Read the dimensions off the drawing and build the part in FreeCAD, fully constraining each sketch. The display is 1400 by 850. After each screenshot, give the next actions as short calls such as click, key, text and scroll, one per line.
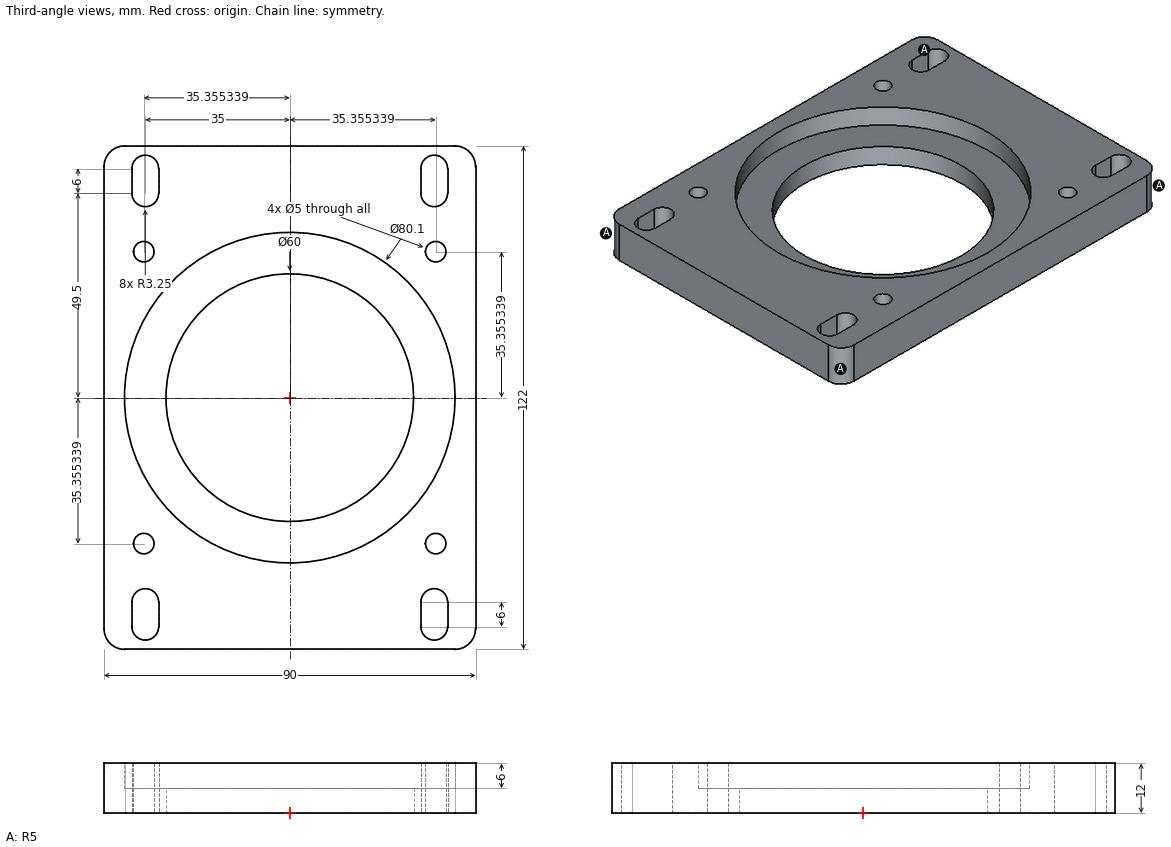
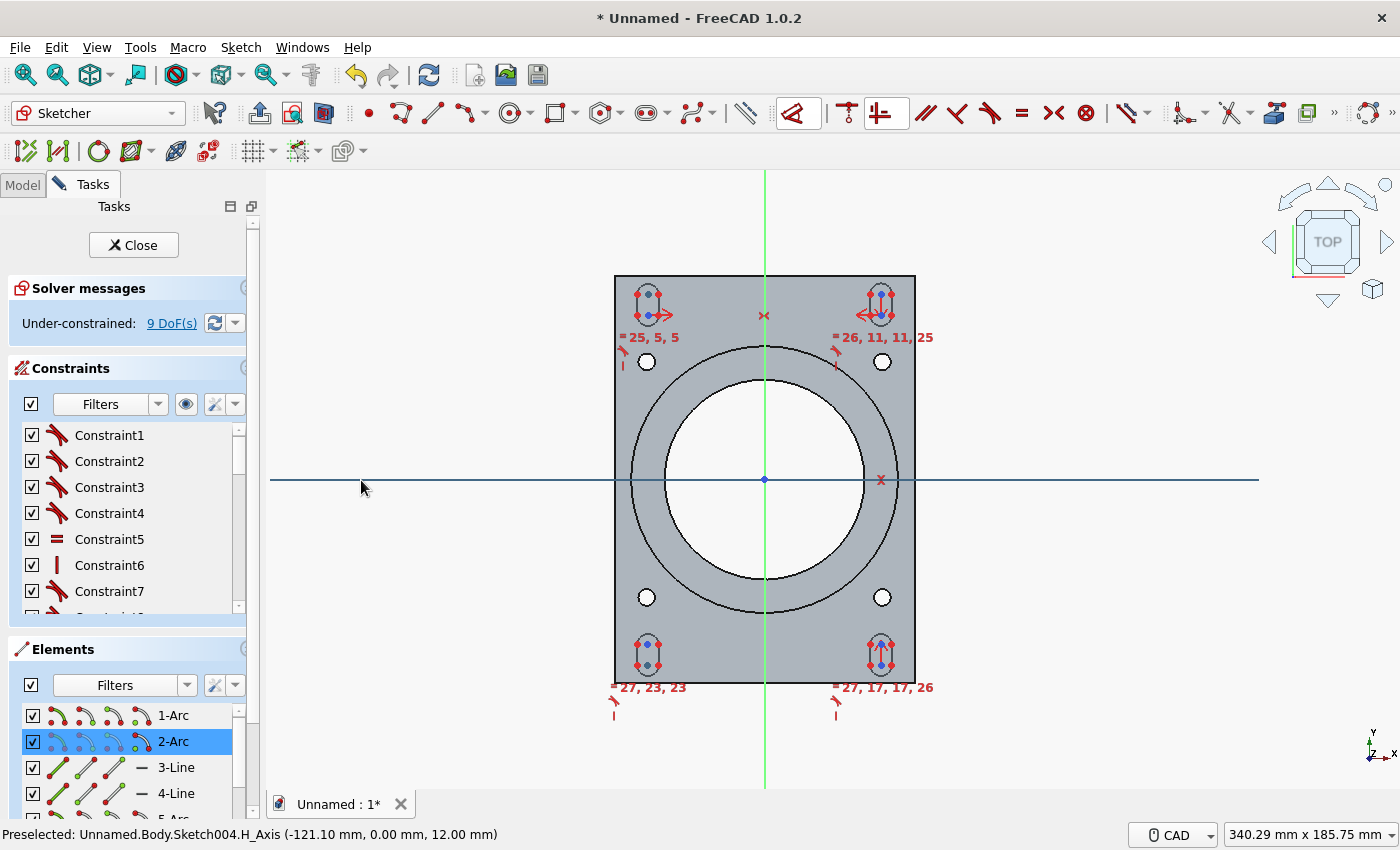
click(1054, 114)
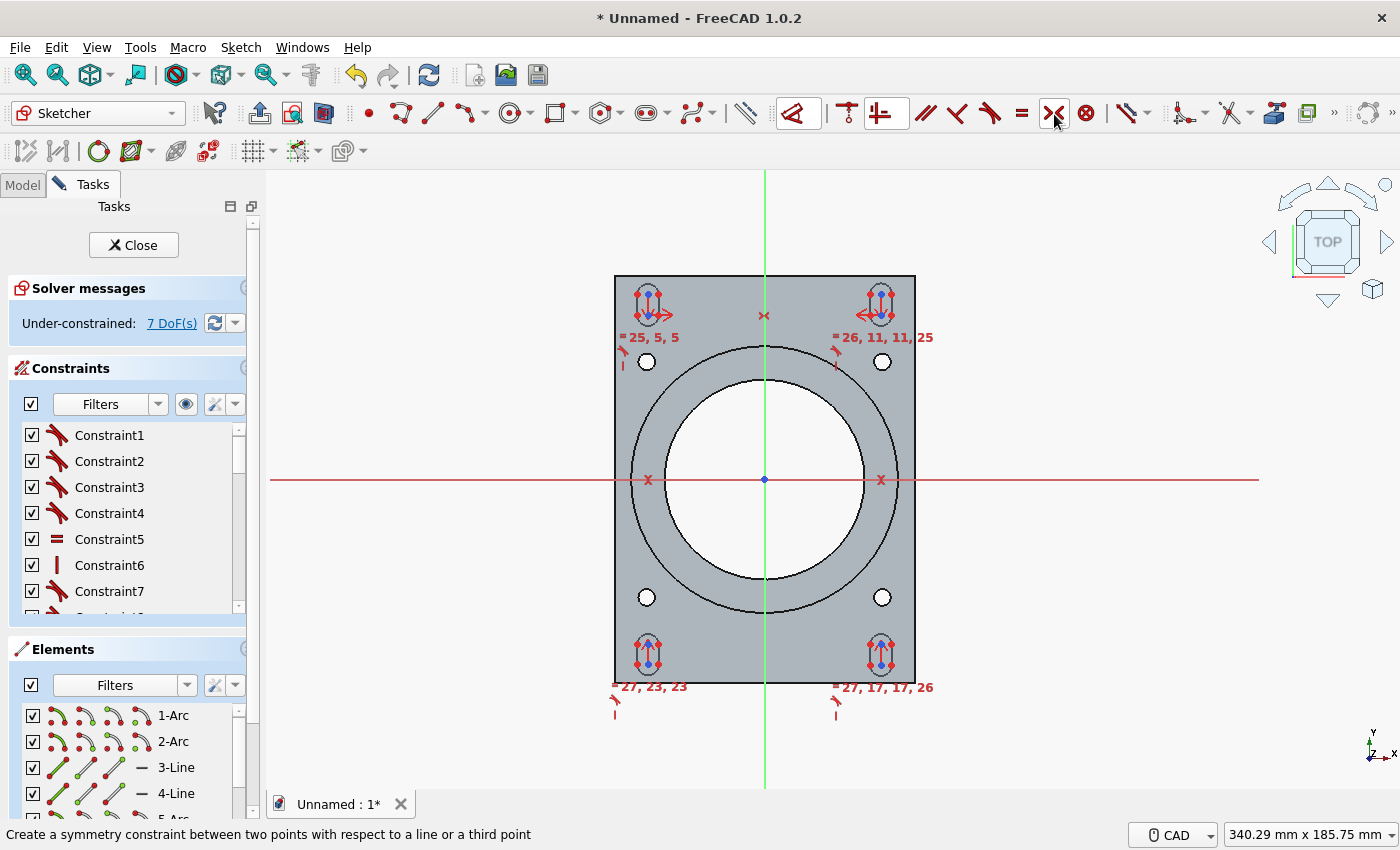
scroll(642, 324, up, 7)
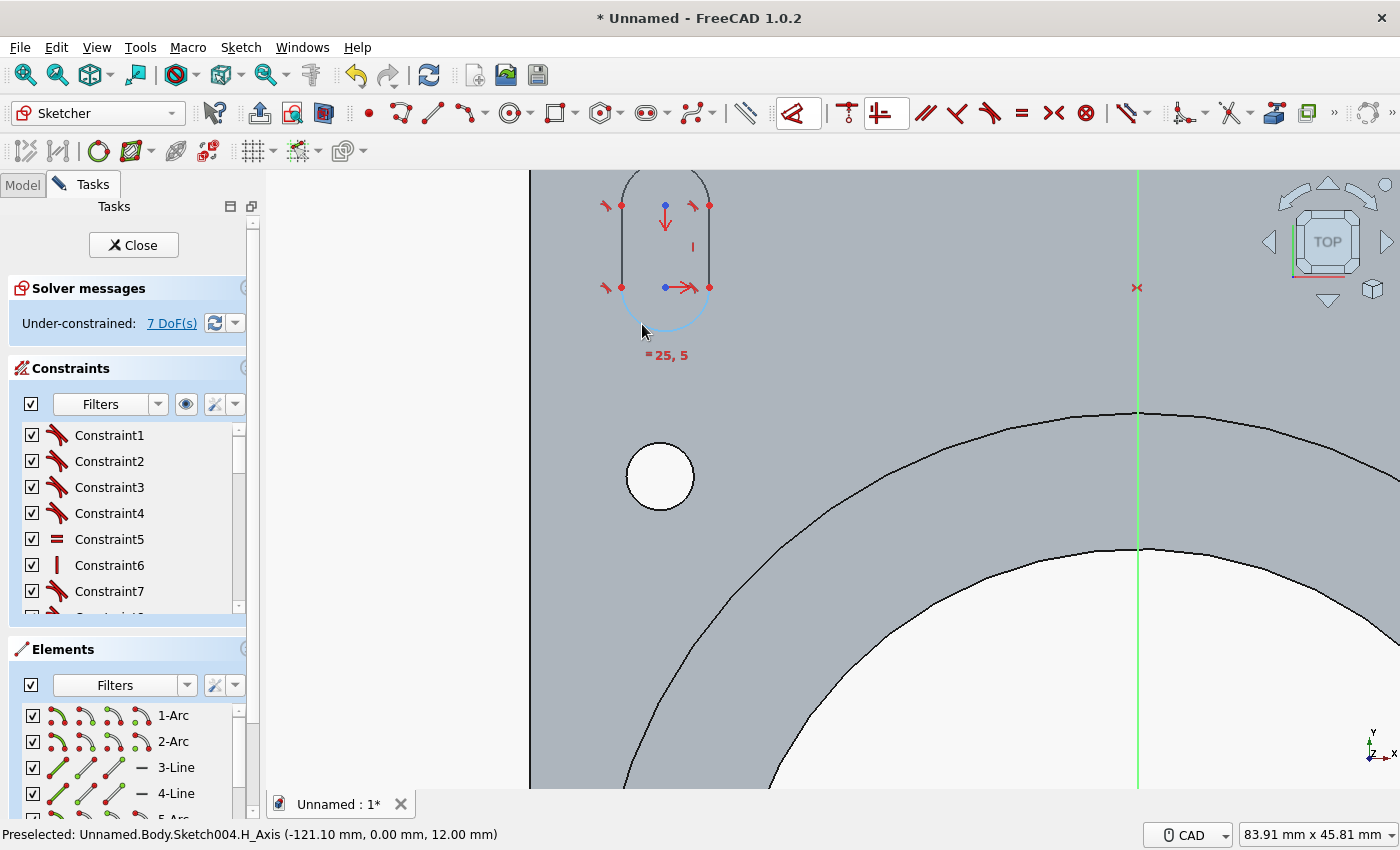
click(640, 323)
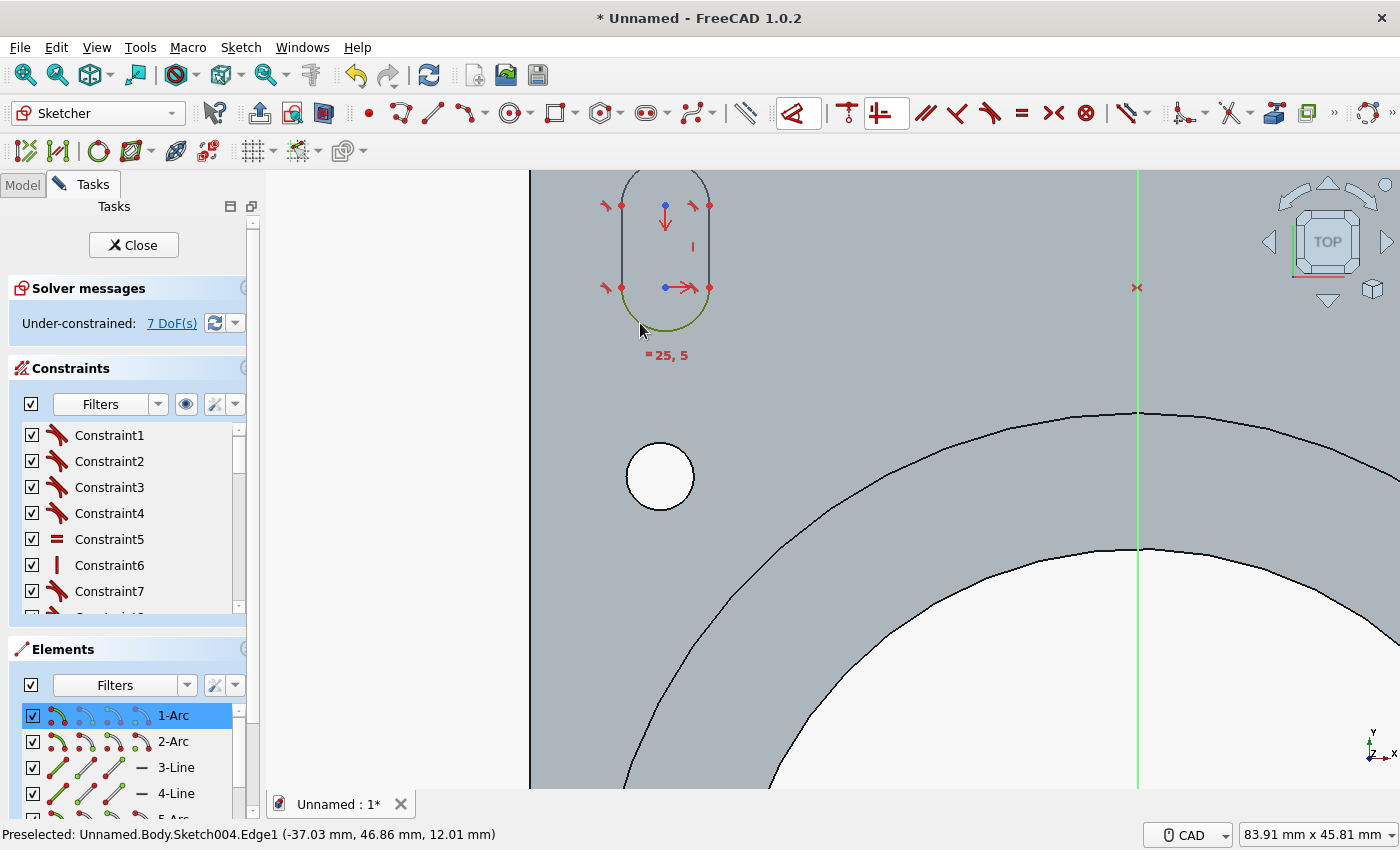
key(k)
key(r)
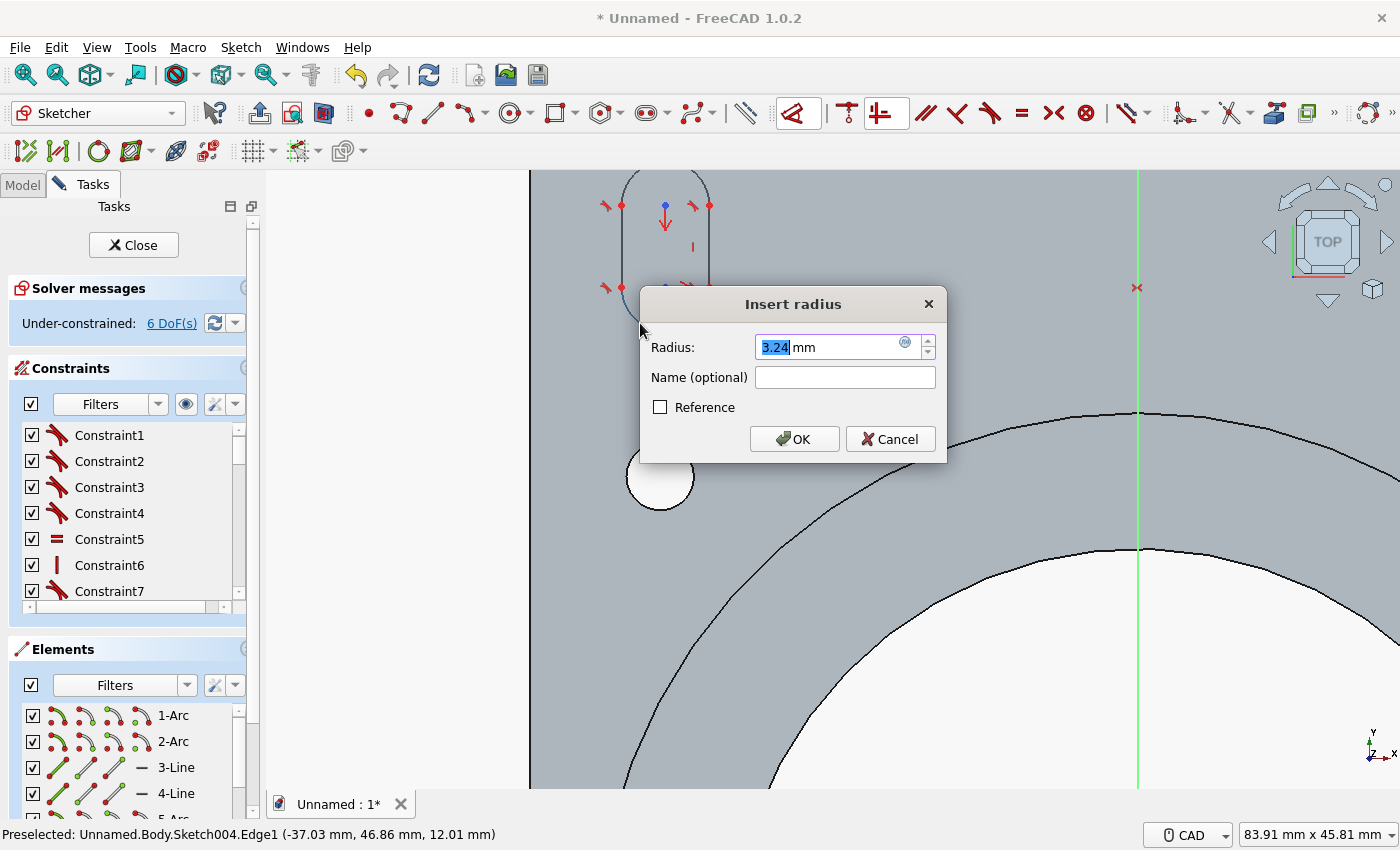
text(3.25)
key(Return)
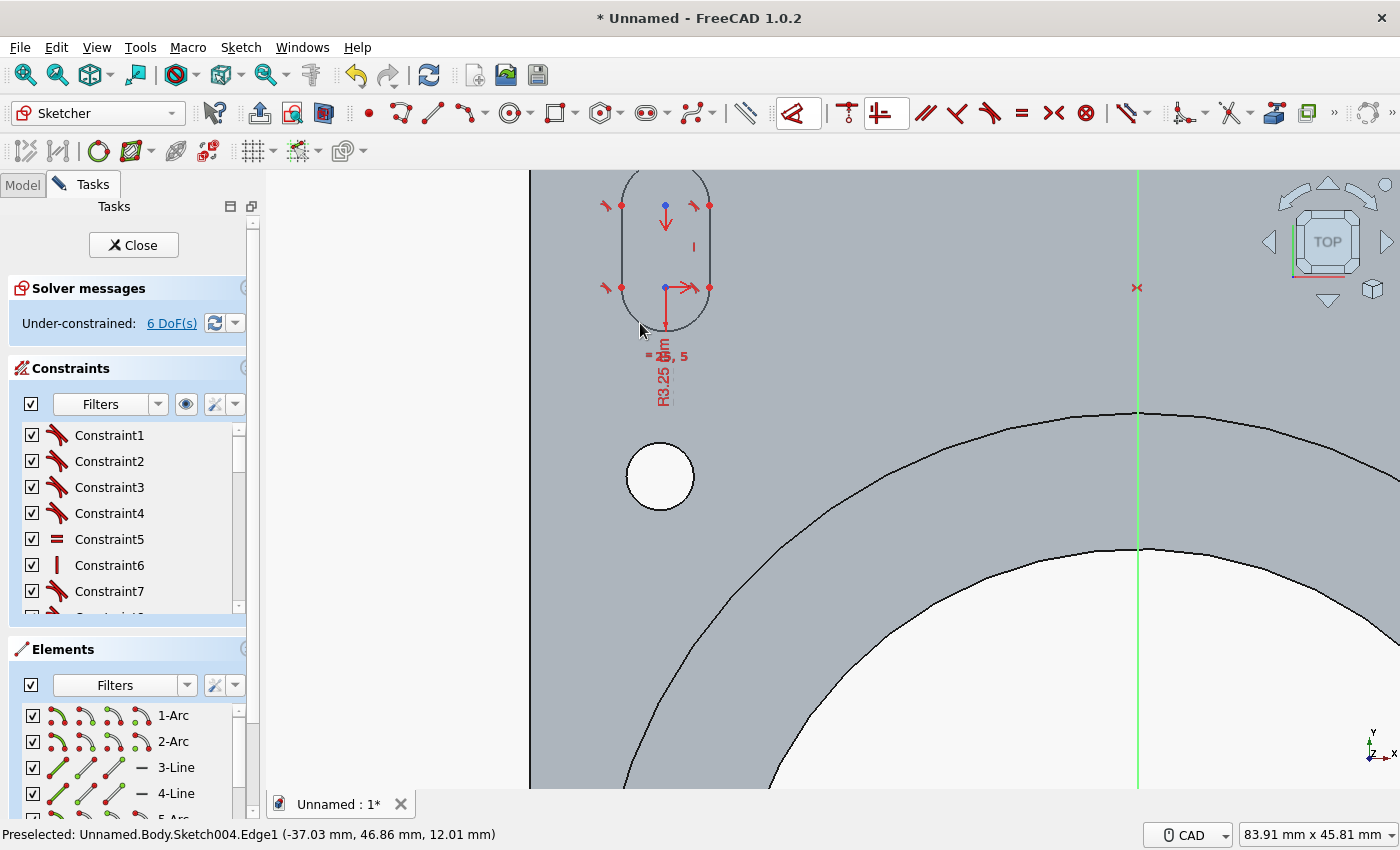
click(622, 263)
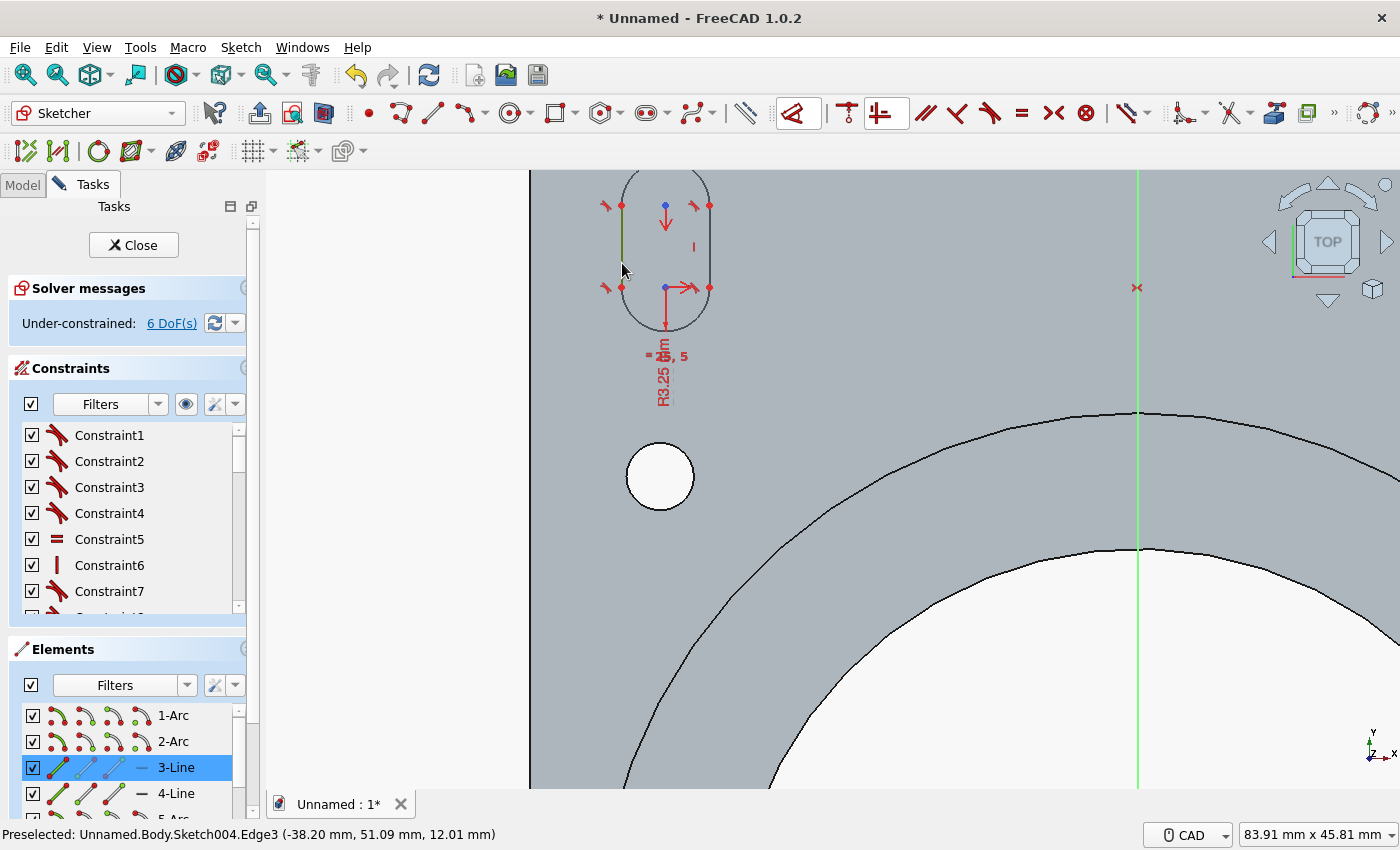
click(816, 114)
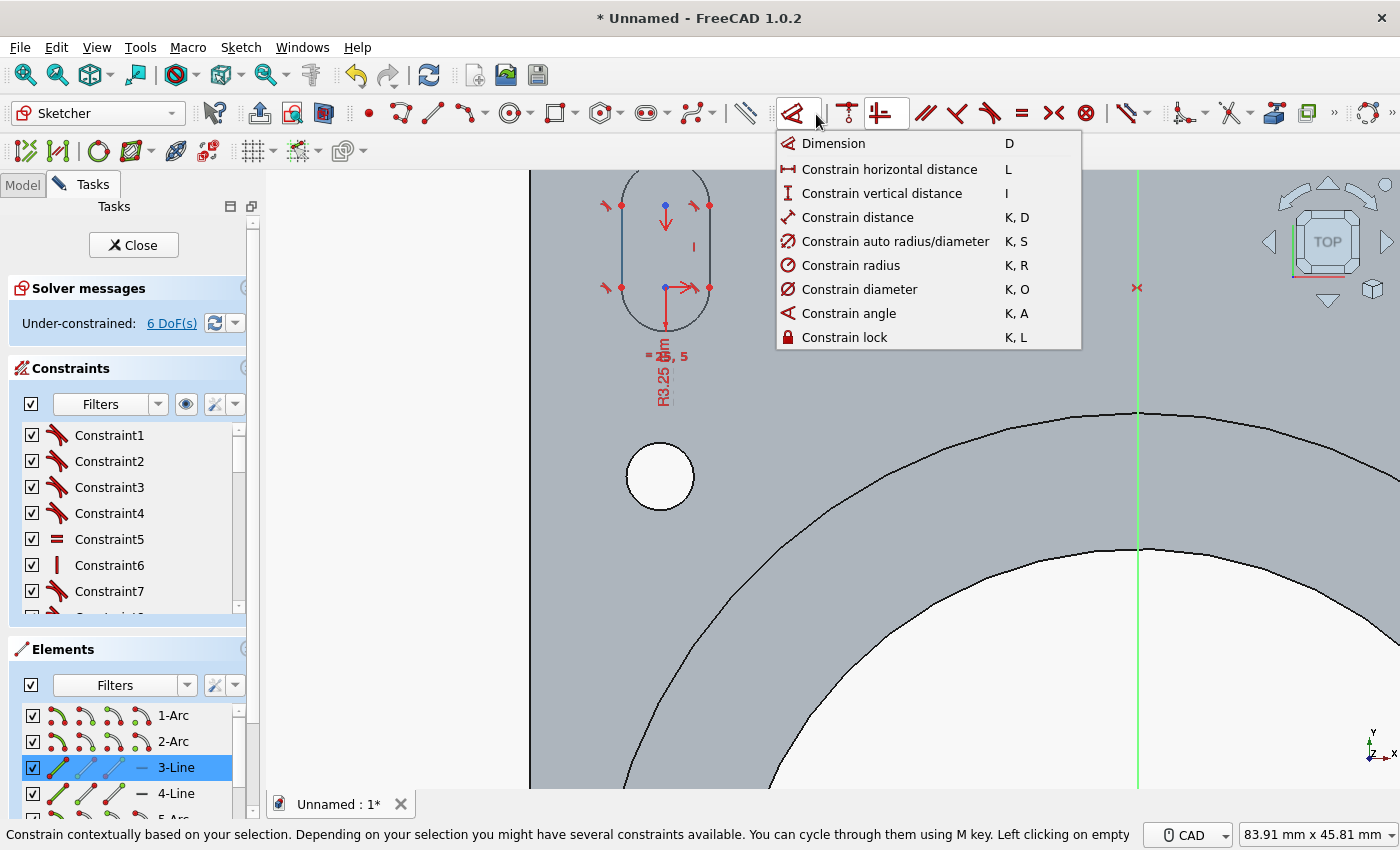
click(929, 193)